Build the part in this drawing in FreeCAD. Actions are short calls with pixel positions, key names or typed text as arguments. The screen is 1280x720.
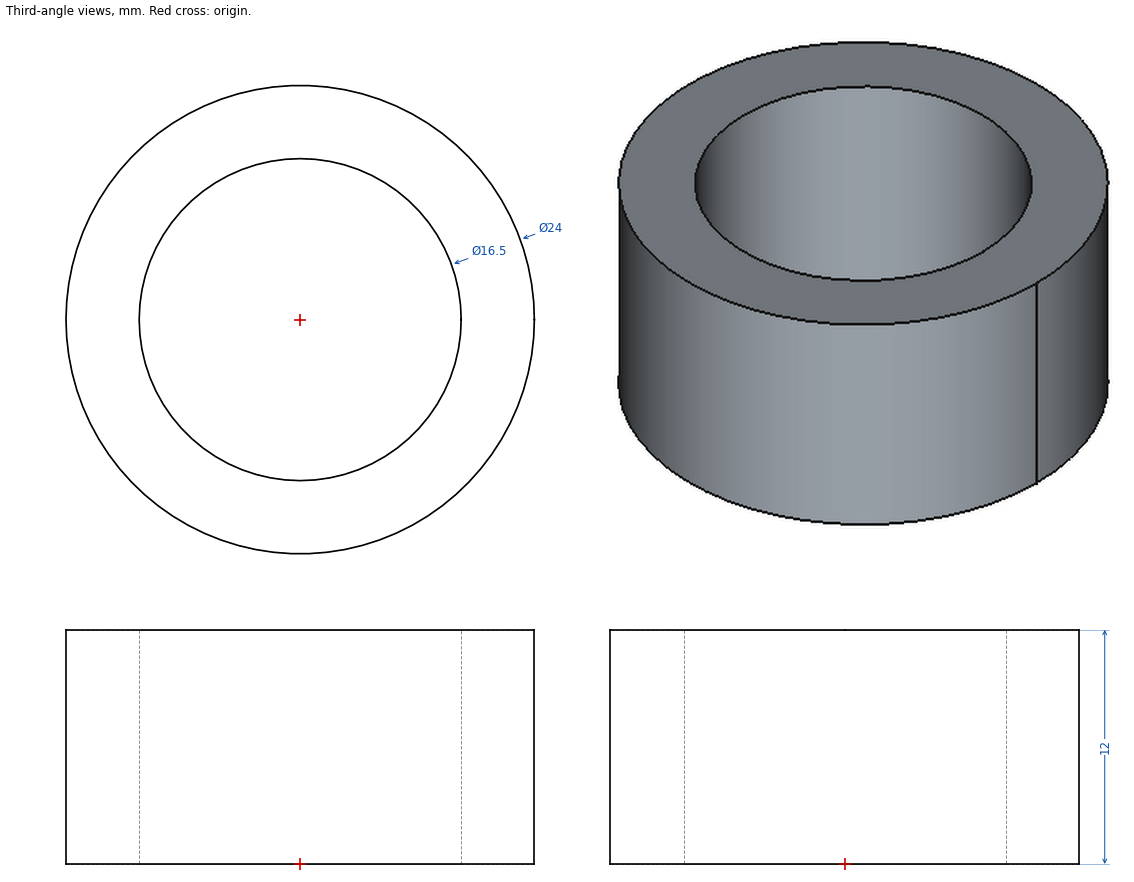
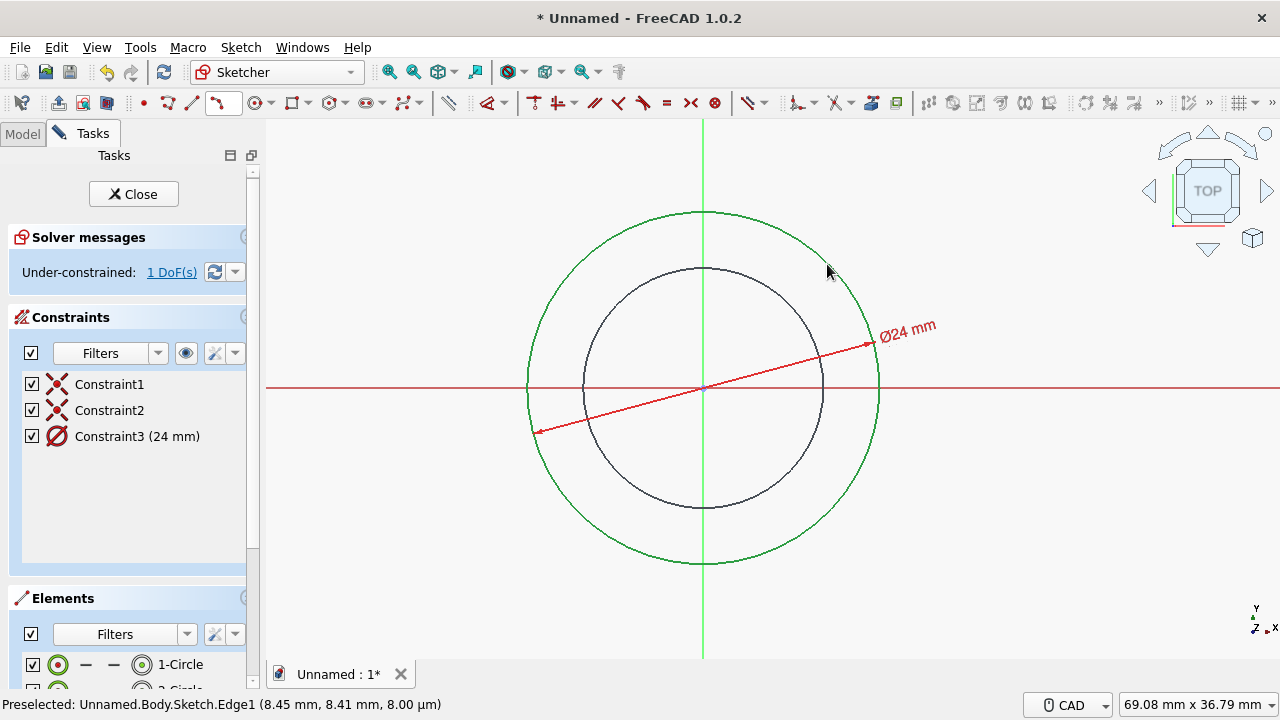
click(788, 303)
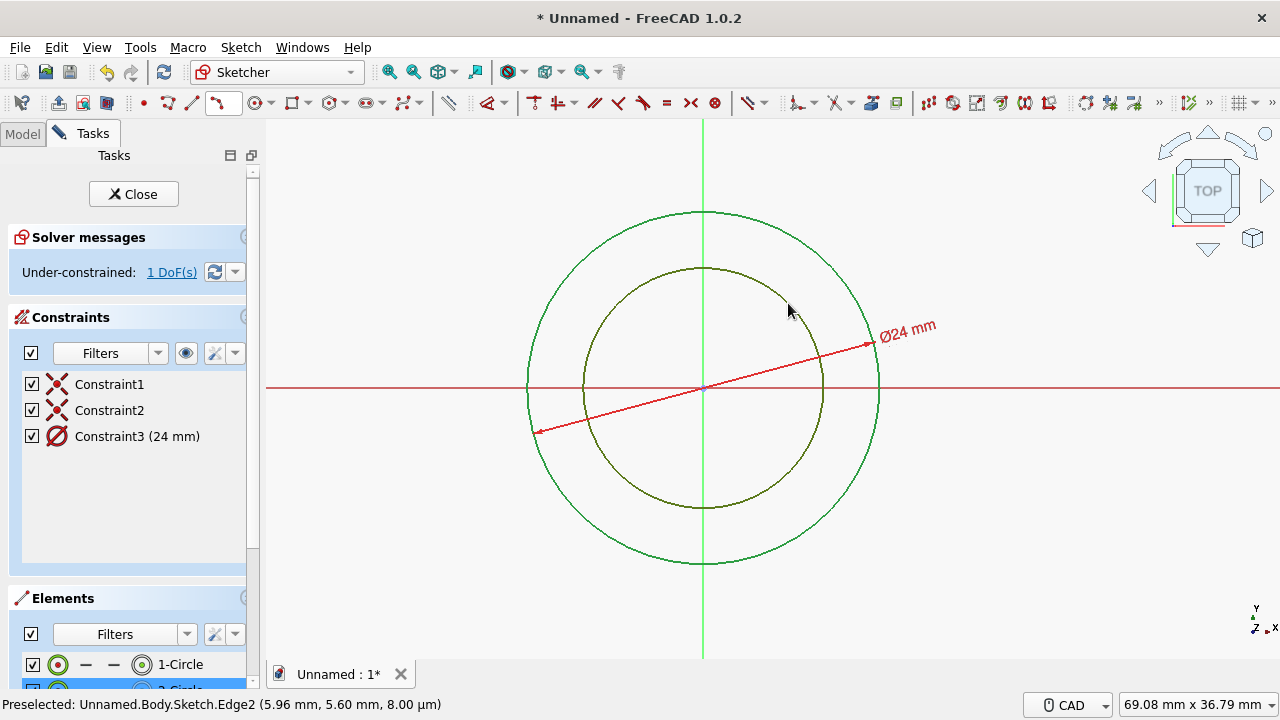
key(k)
key(o)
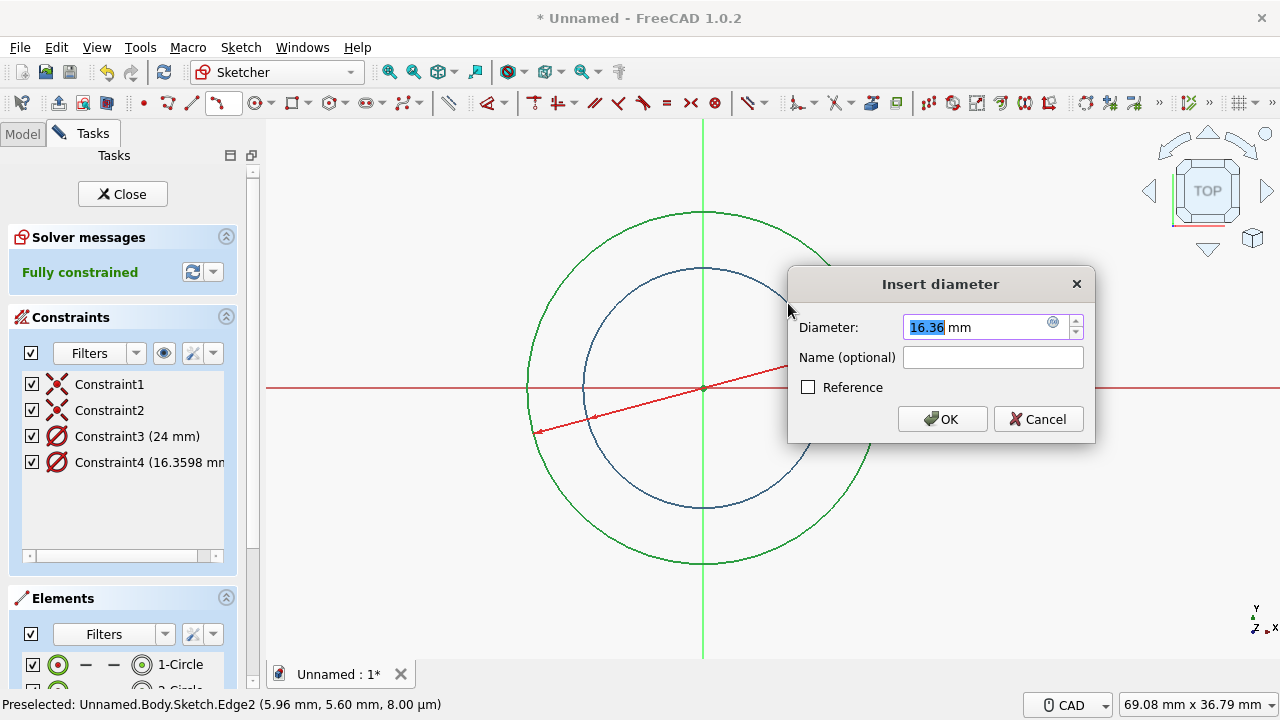
text(16.5)
key(Return)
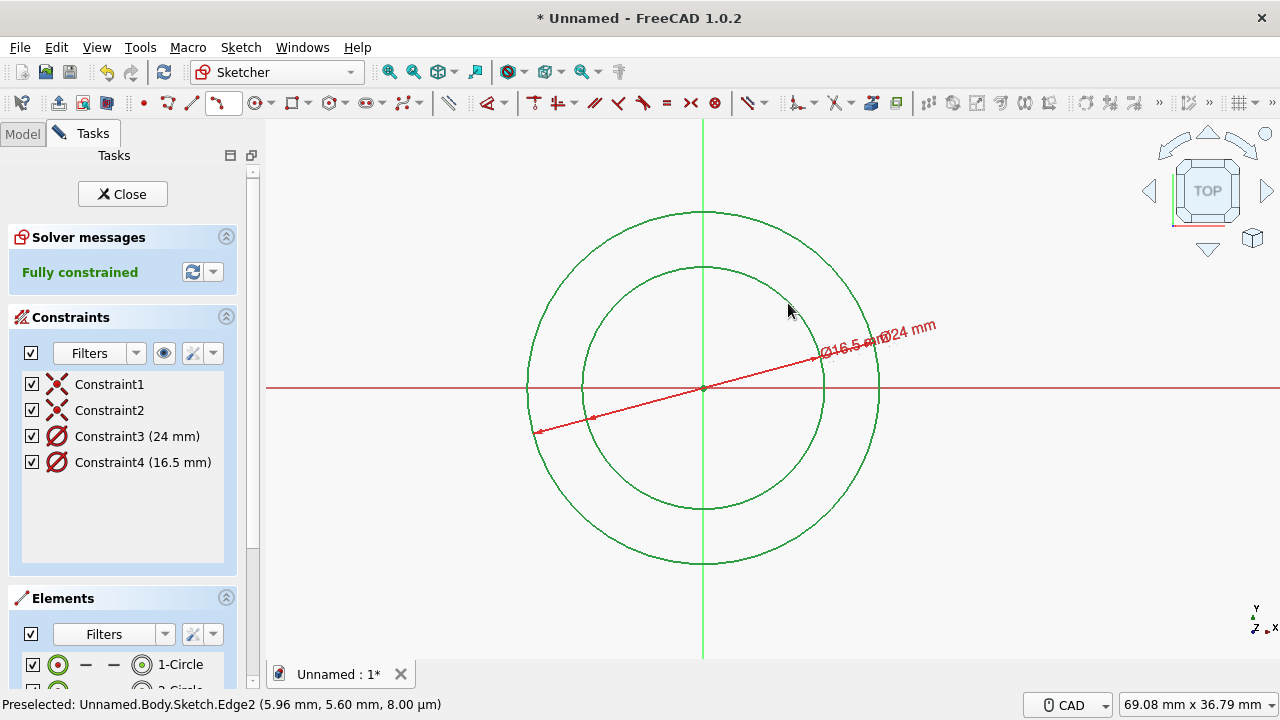
click(123, 194)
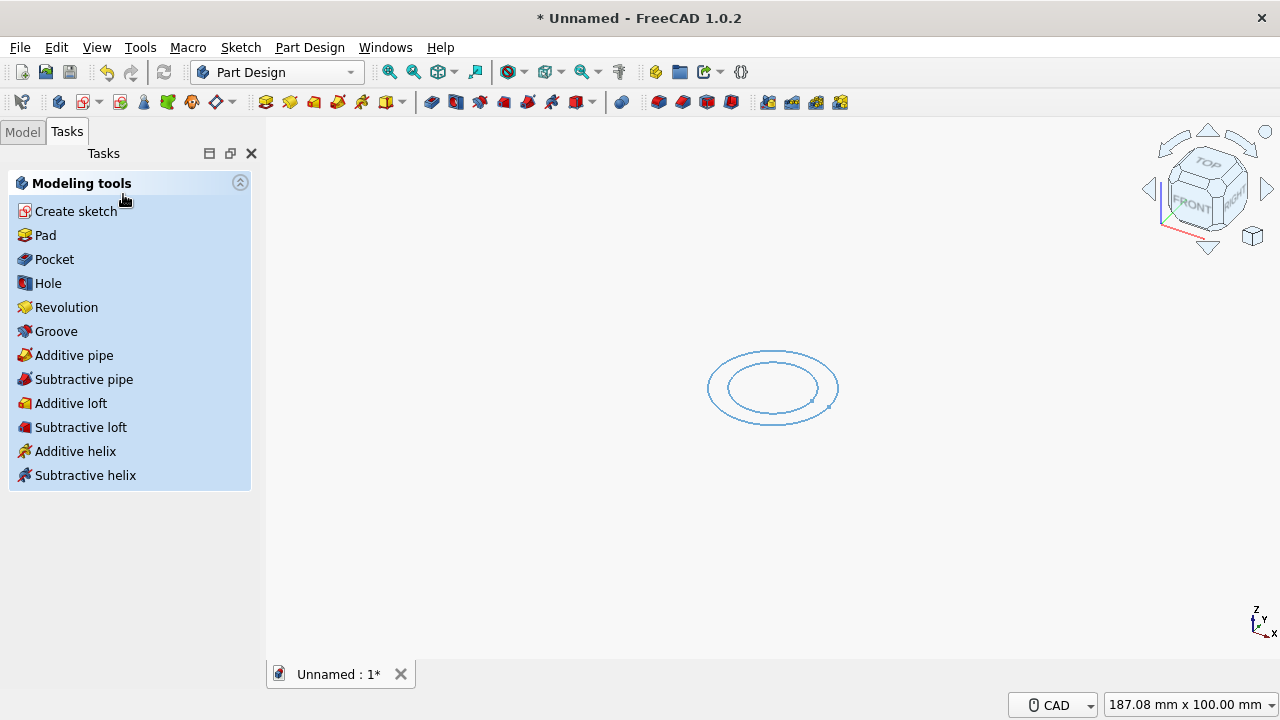
click(266, 102)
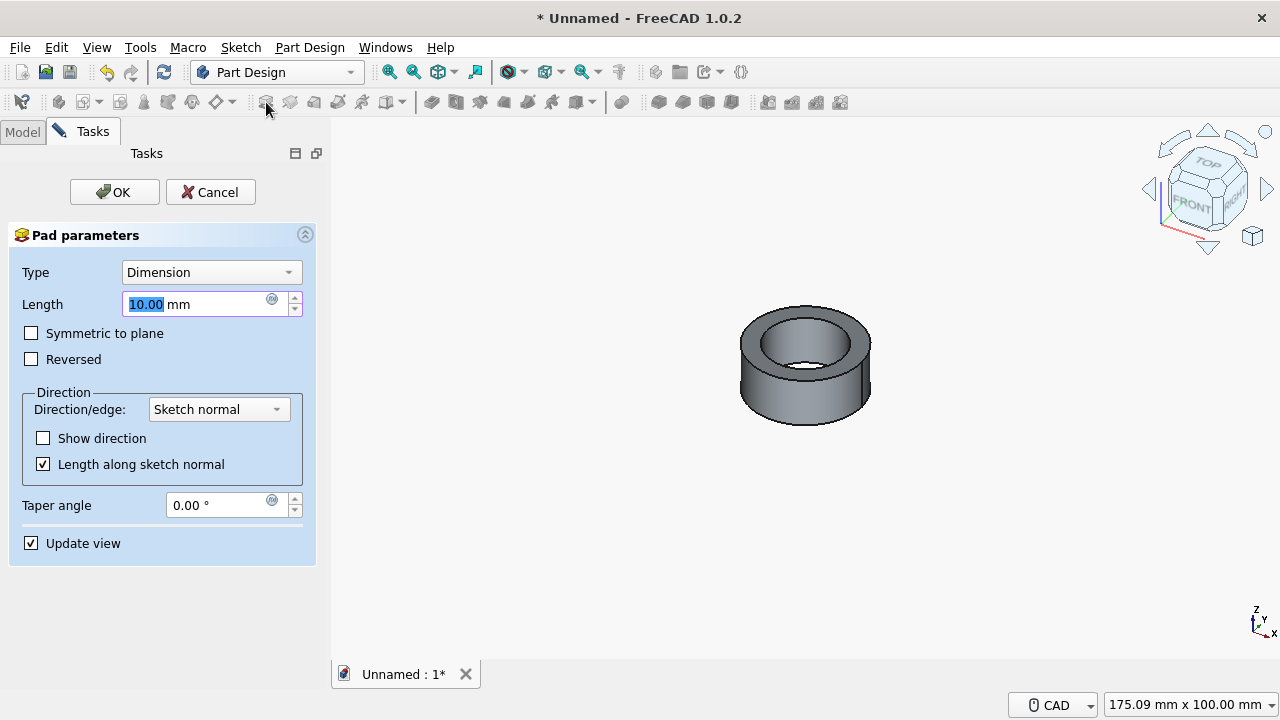
text(12)
key(Tab)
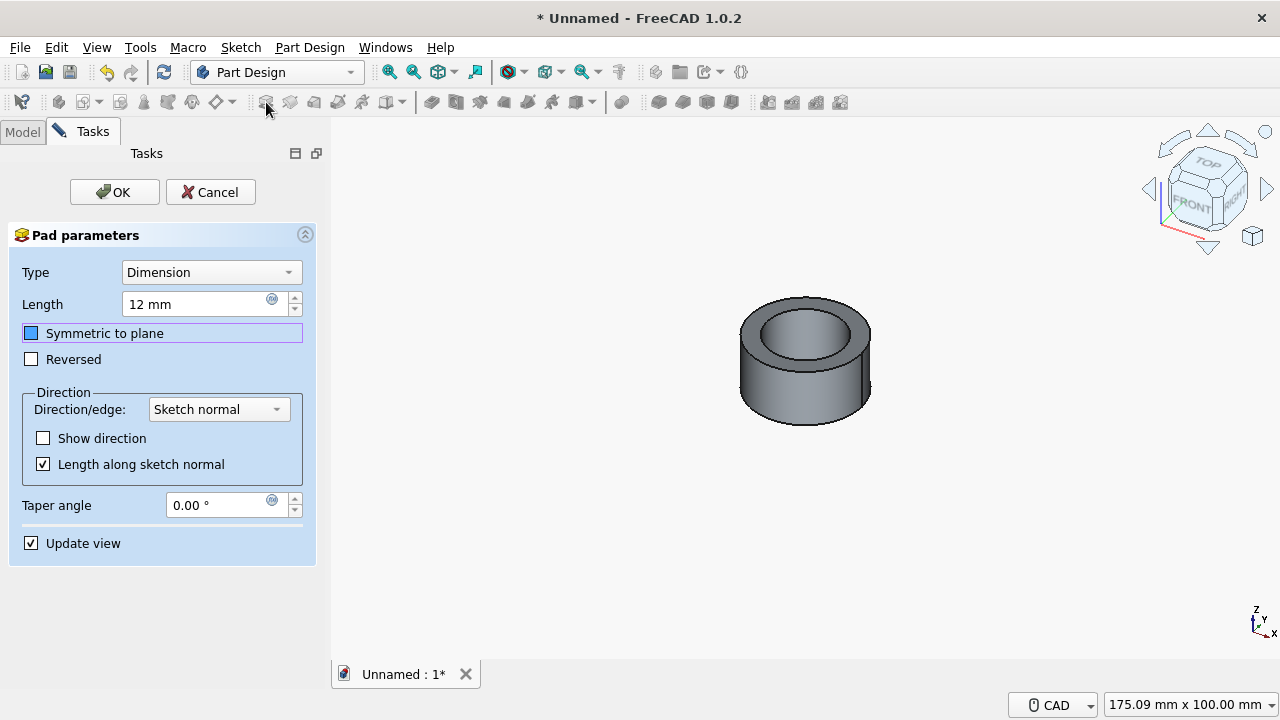
click(115, 192)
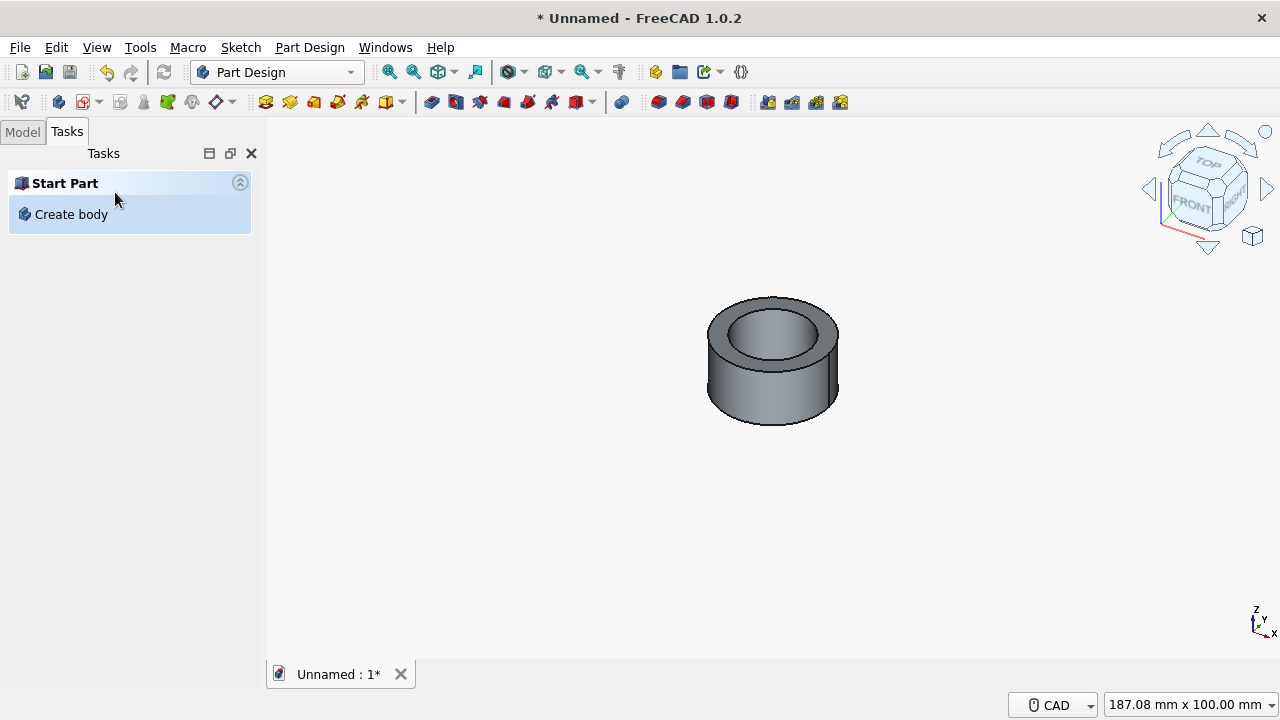
key(0)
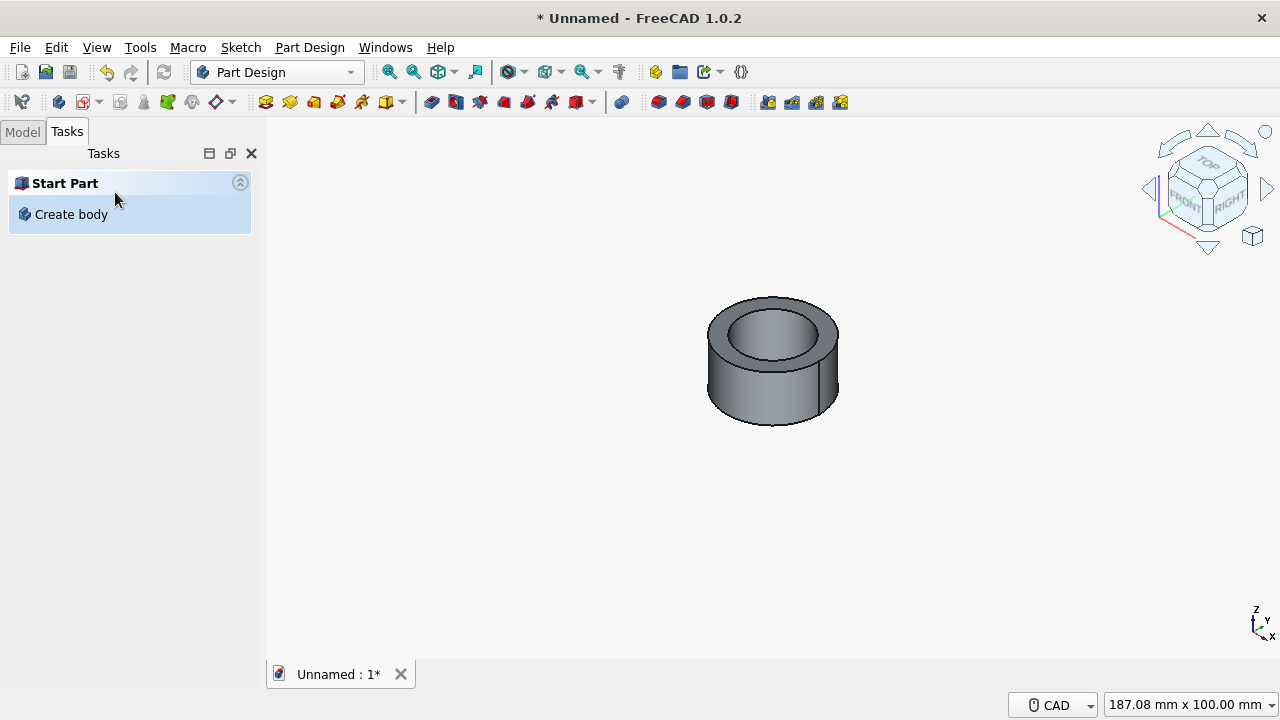
key(v)
key(f)